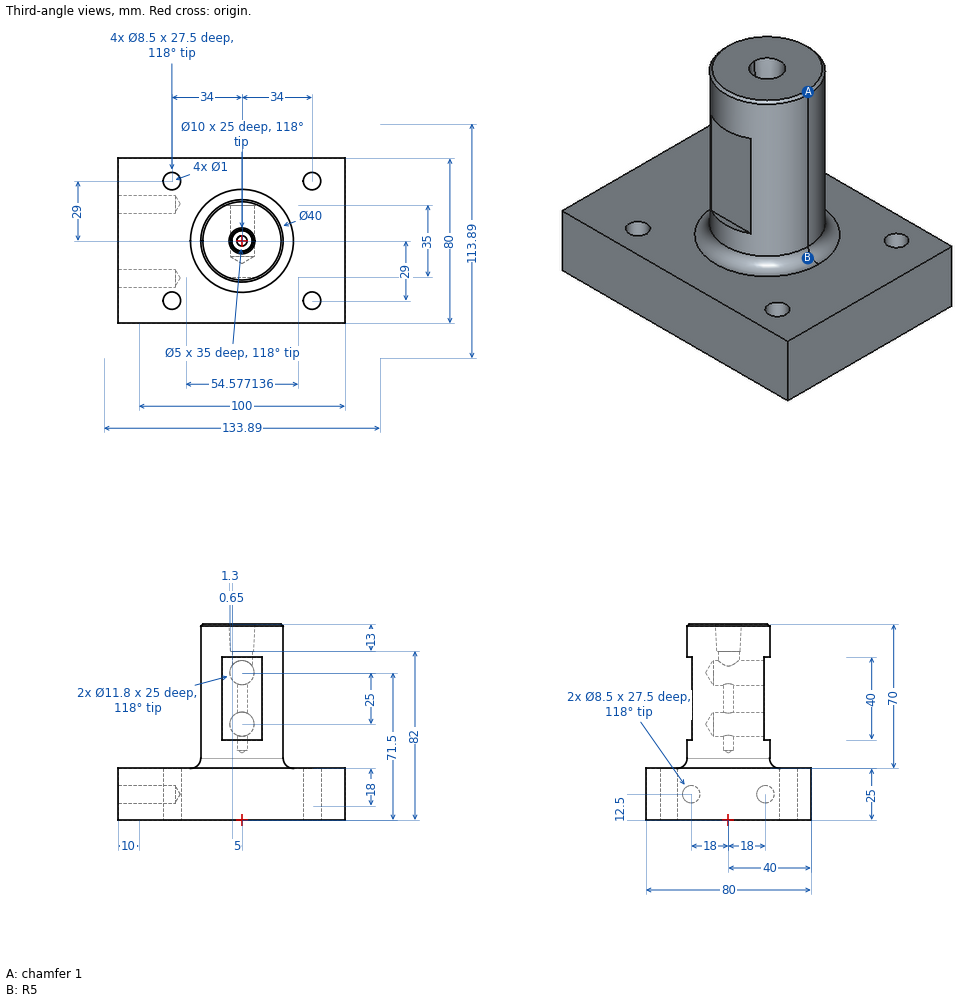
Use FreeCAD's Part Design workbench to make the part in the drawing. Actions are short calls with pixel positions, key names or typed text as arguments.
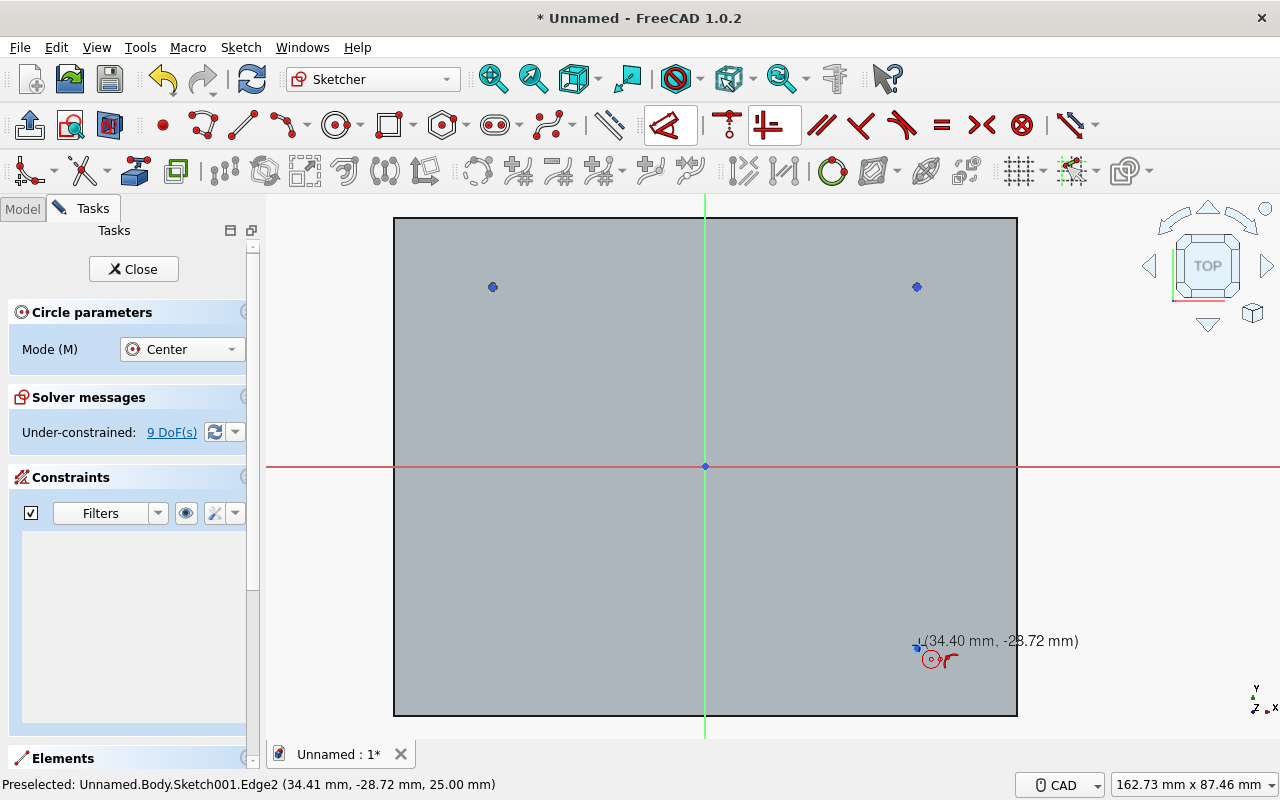
scroll(493, 648, up, 10)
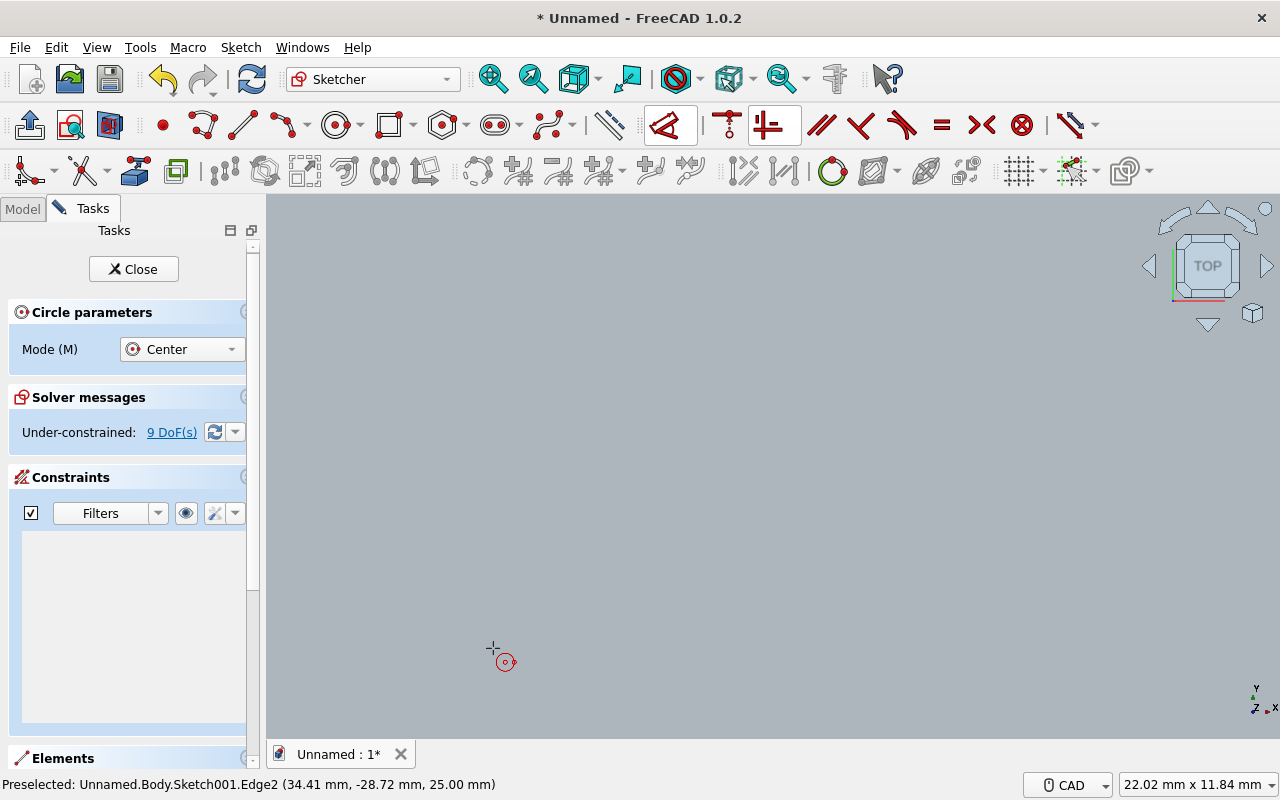
scroll(492, 648, down, 10)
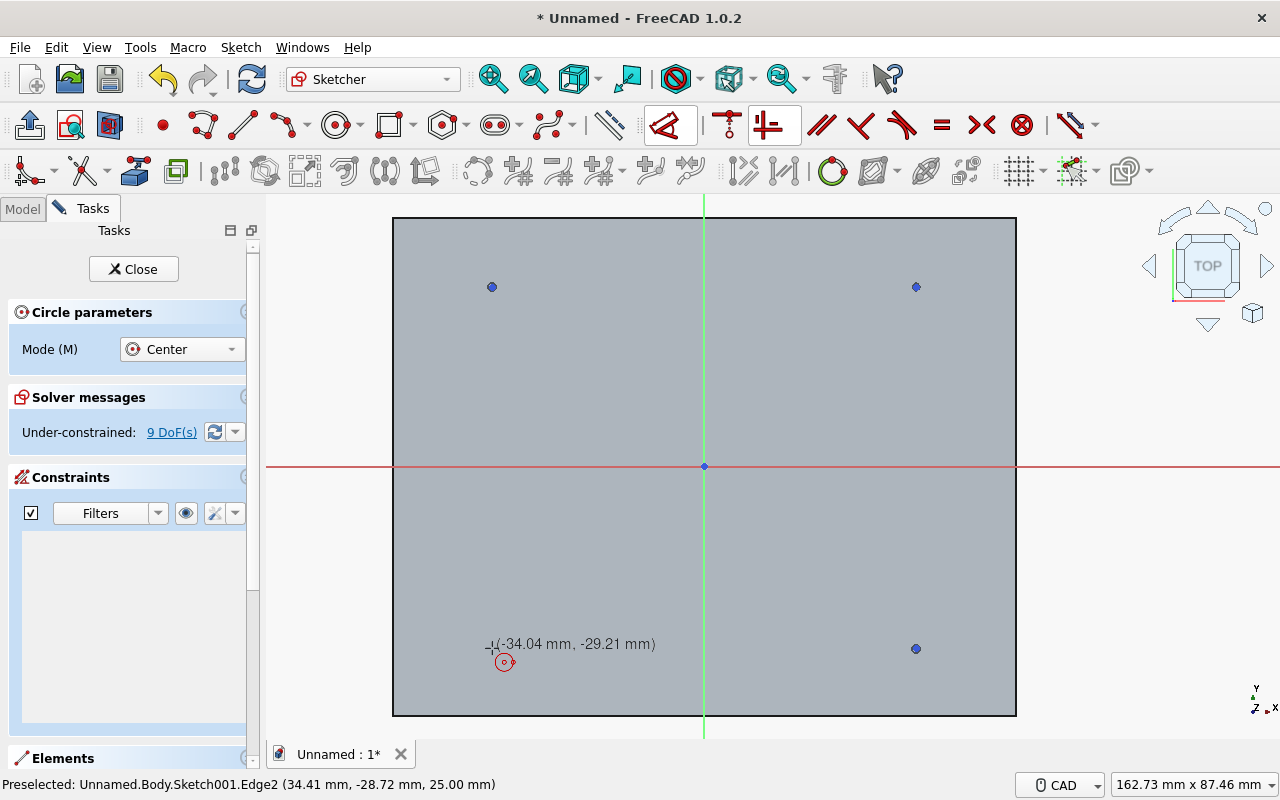
click(492, 648)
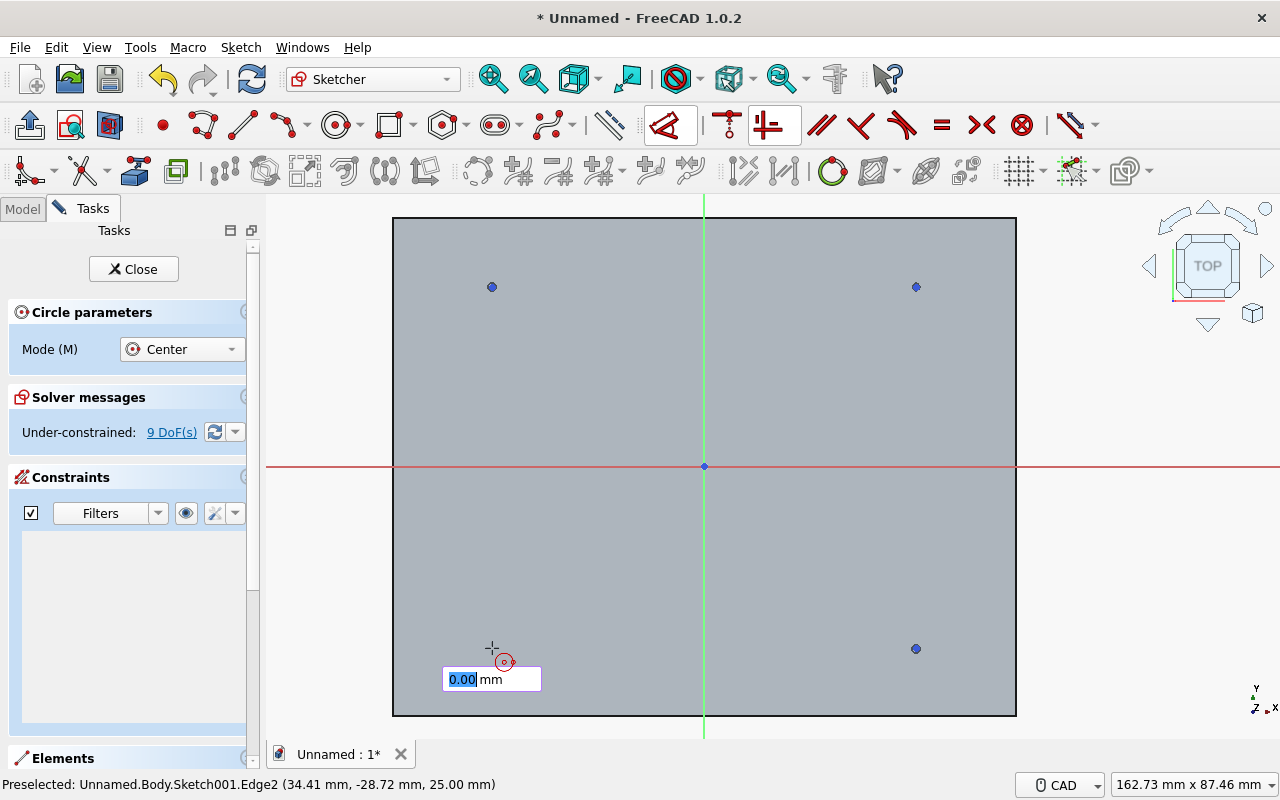
scroll(495, 645, up, 9)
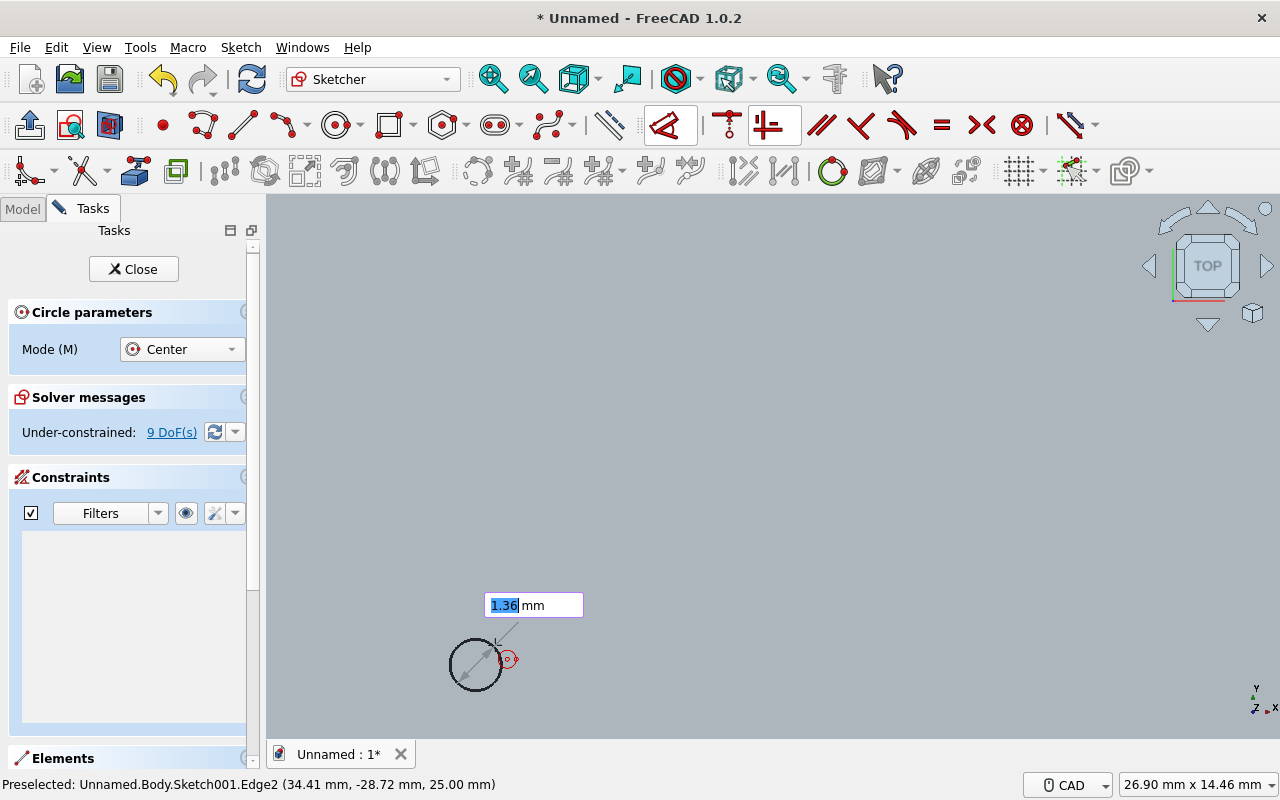
click(492, 643)
key(Escape)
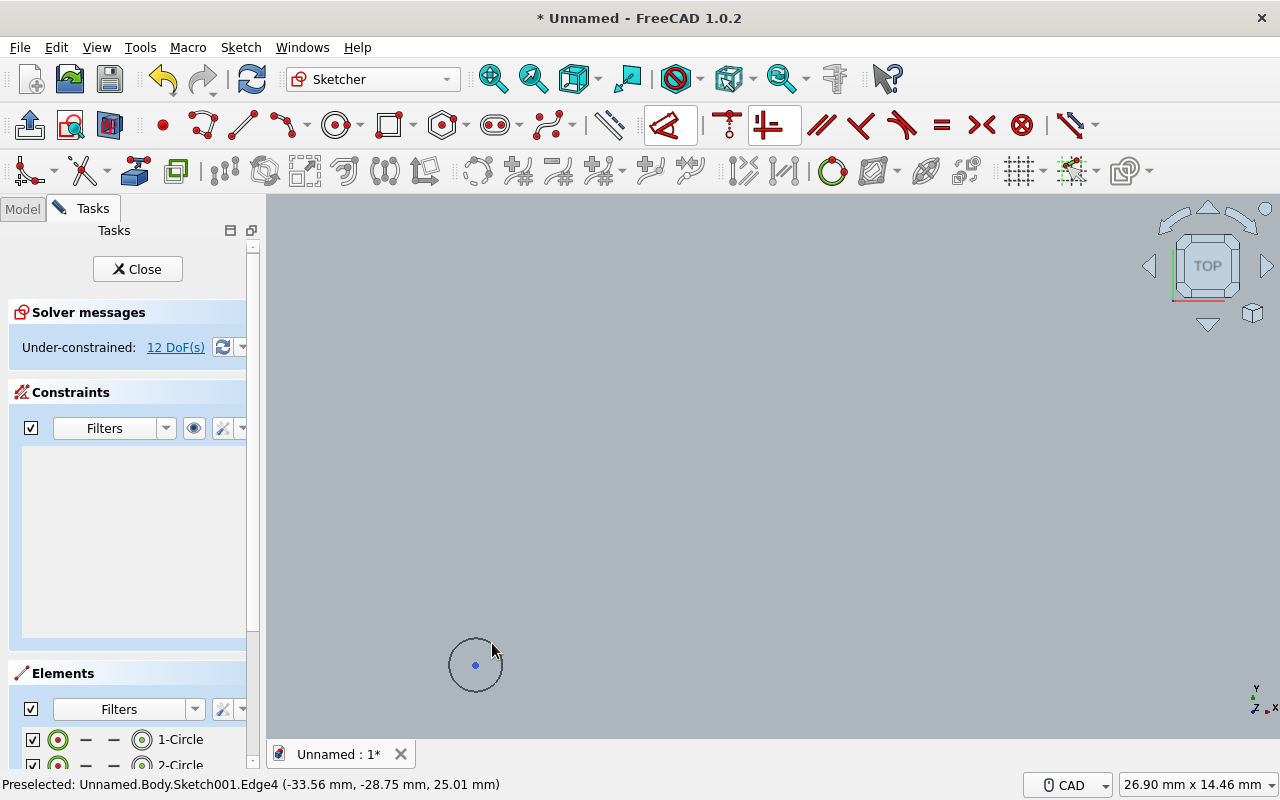
scroll(495, 645, down, 9)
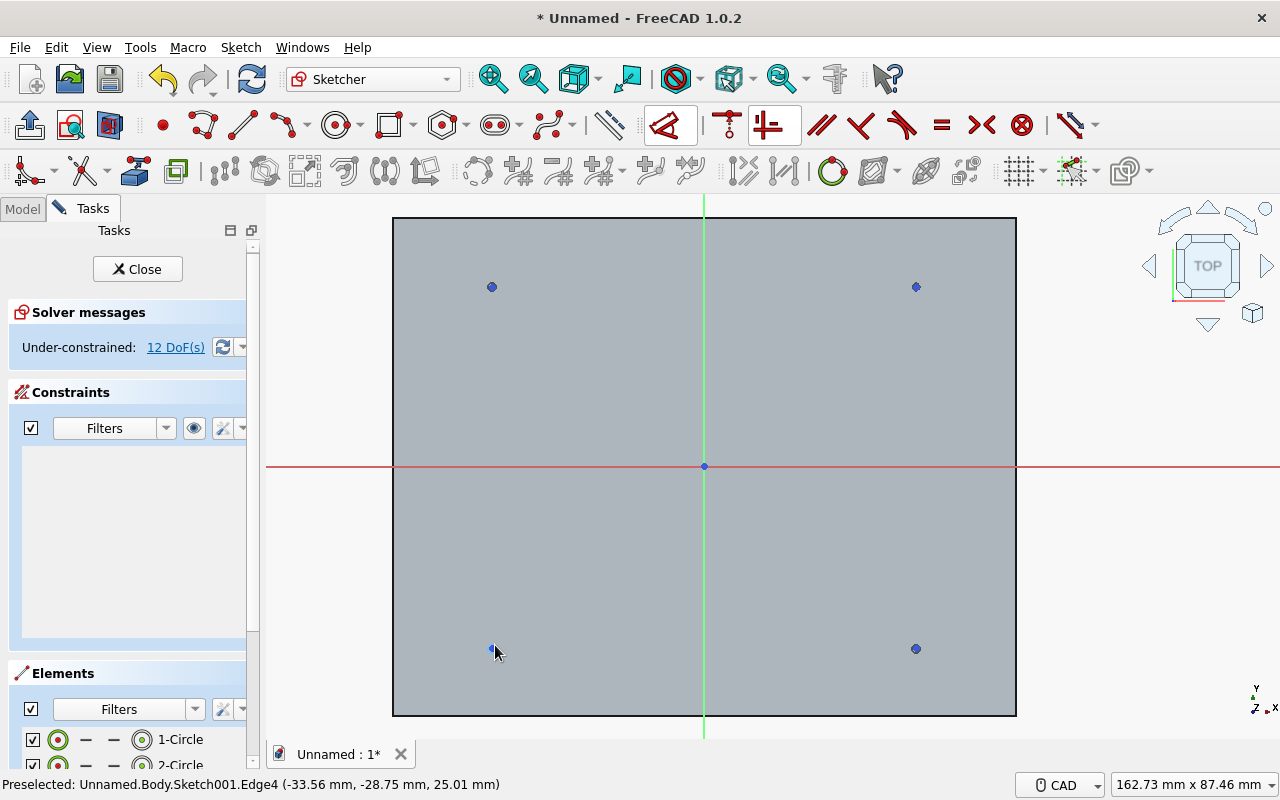
scroll(495, 284, up, 7)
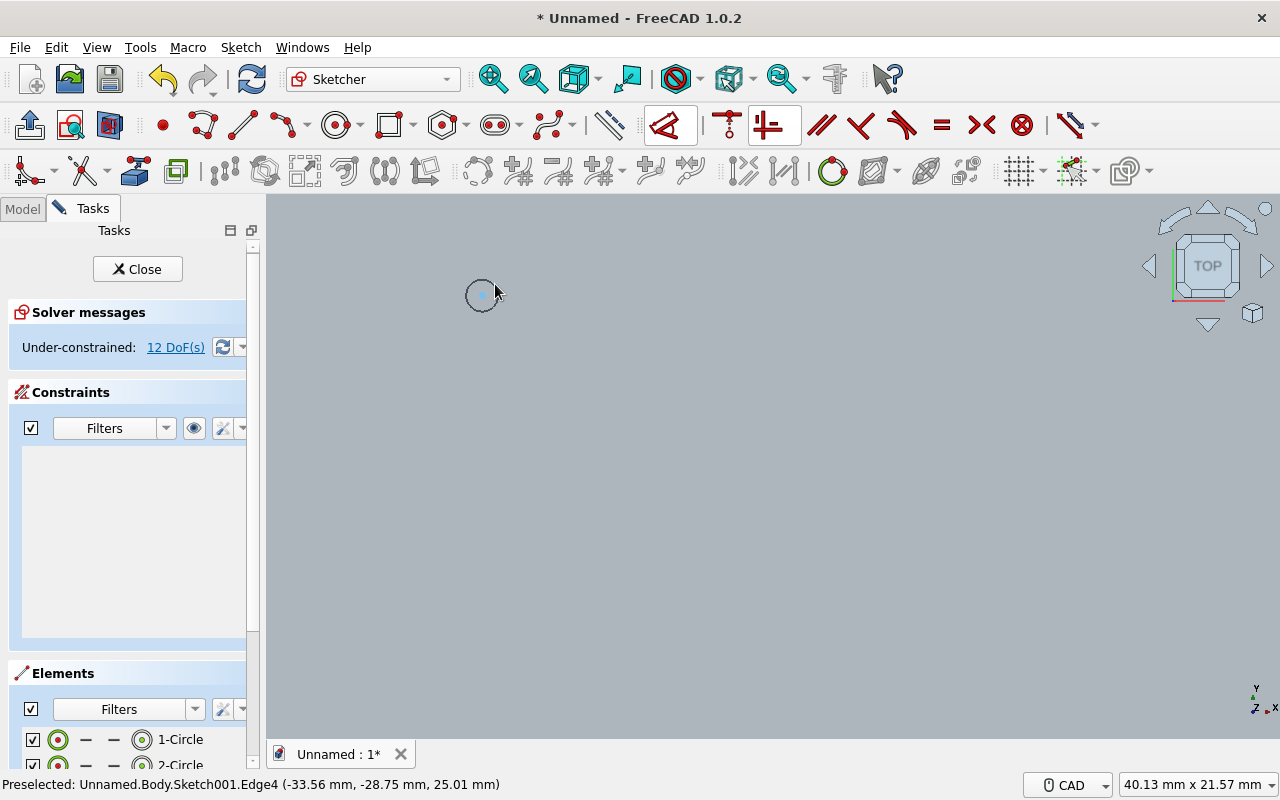
click(493, 284)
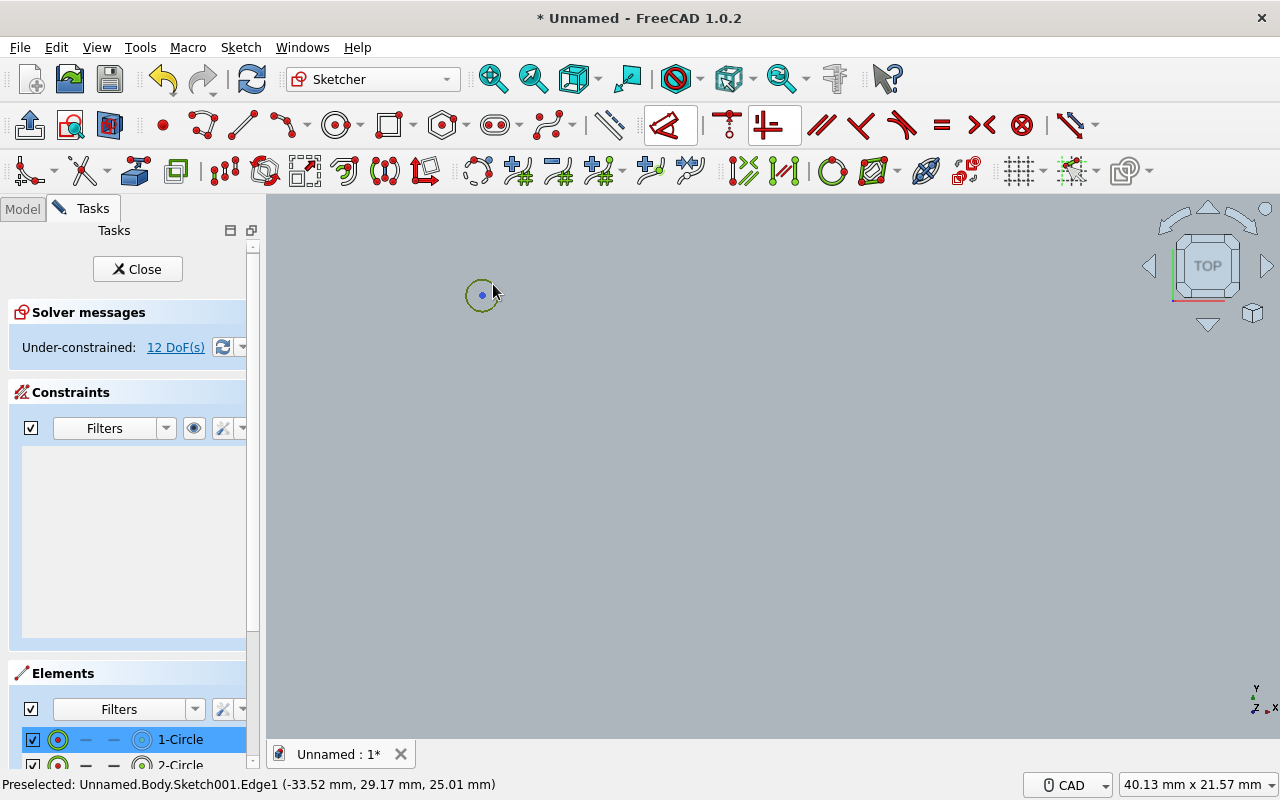
scroll(495, 284, down, 7)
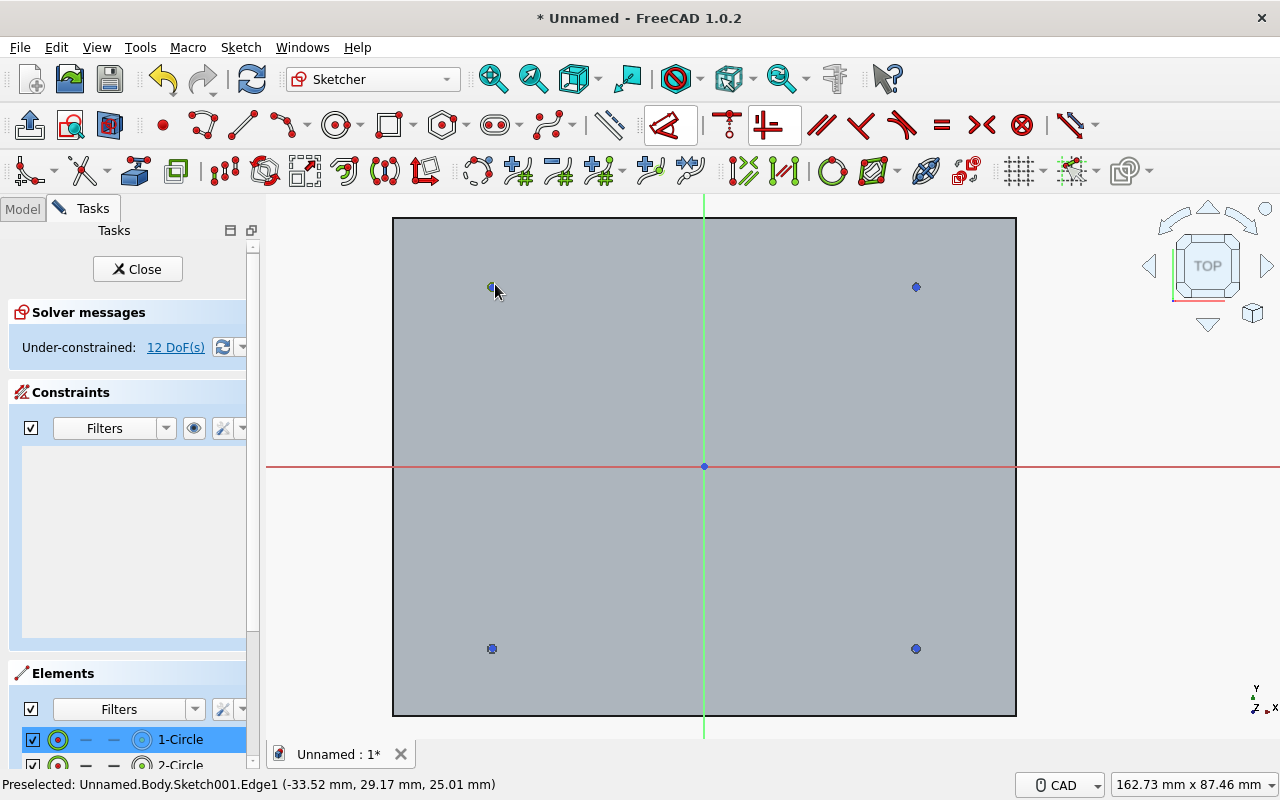
scroll(919, 284, up, 7)